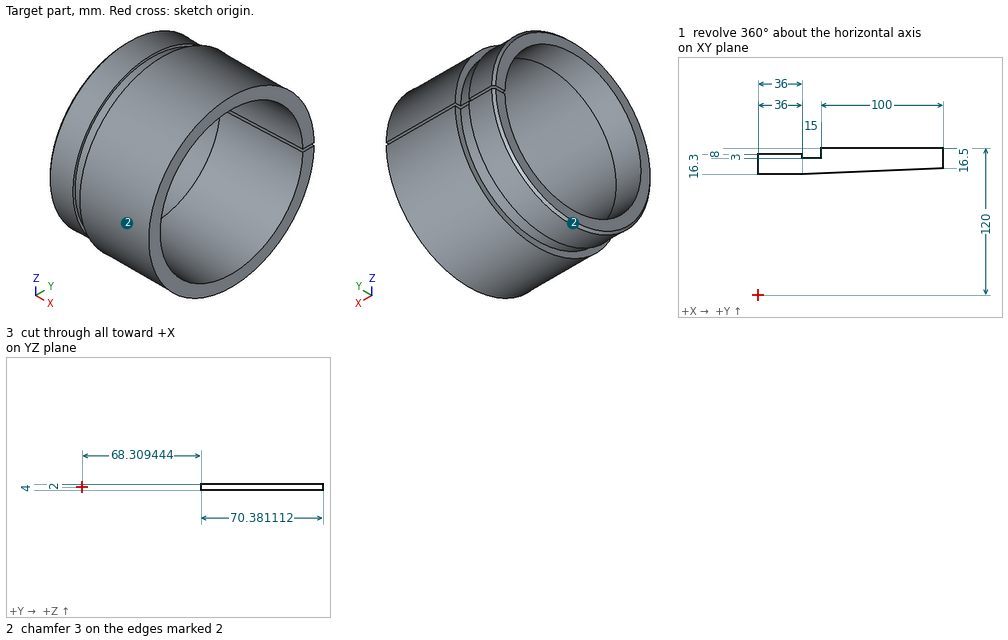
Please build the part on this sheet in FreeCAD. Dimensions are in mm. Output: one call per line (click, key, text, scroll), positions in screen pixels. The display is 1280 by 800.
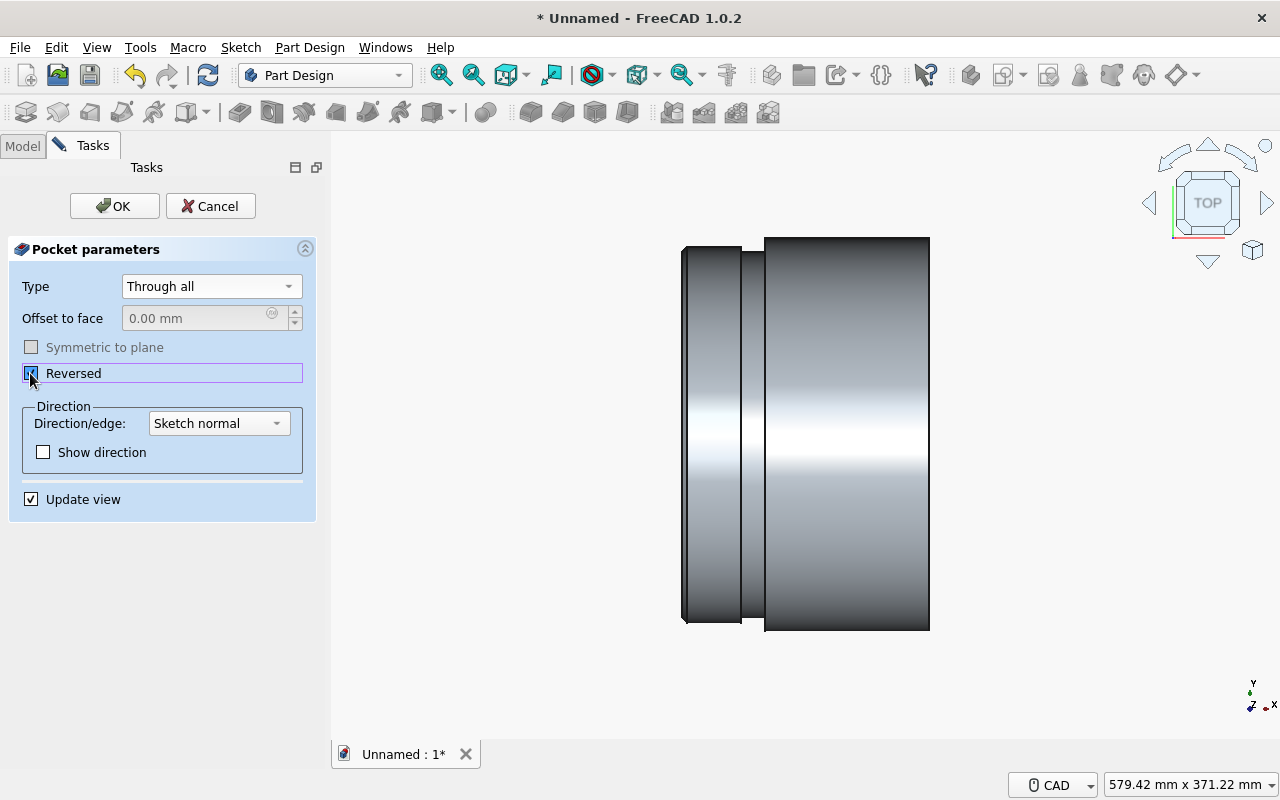
click(115, 206)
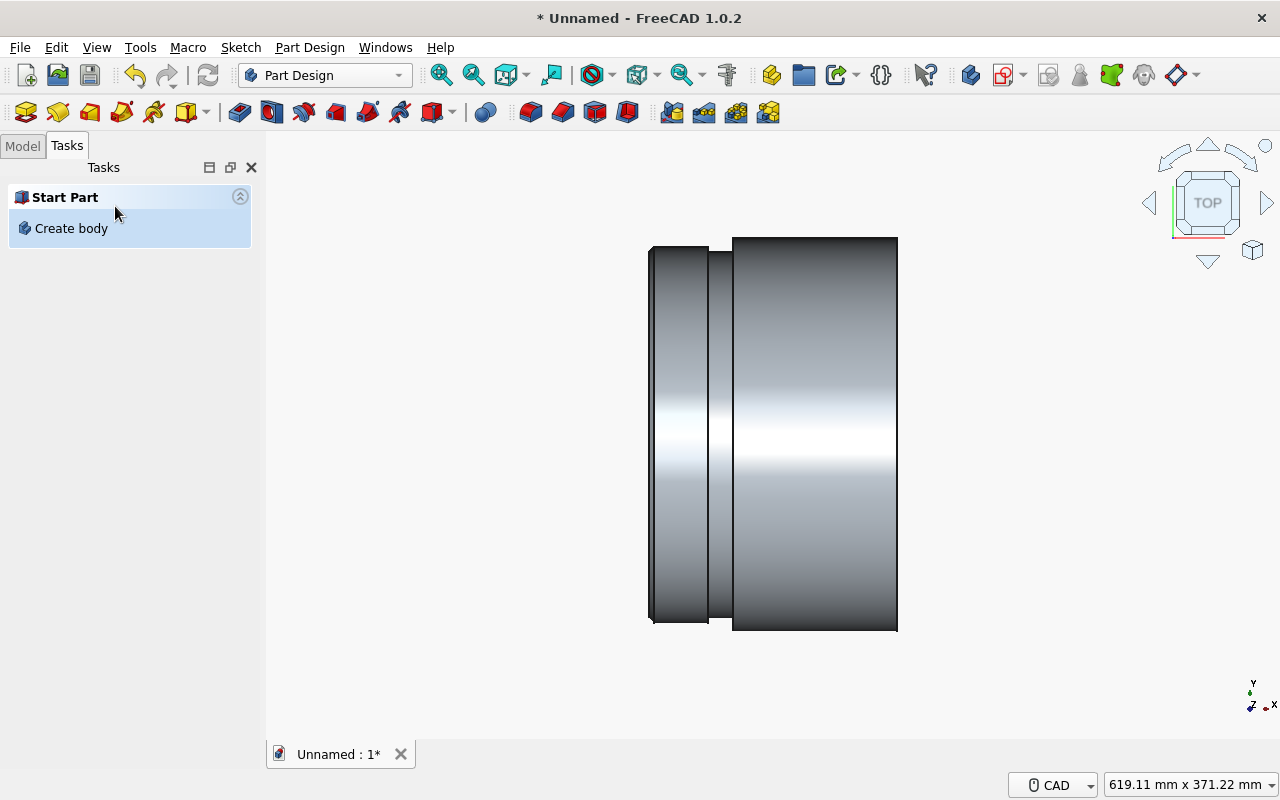
key(0)